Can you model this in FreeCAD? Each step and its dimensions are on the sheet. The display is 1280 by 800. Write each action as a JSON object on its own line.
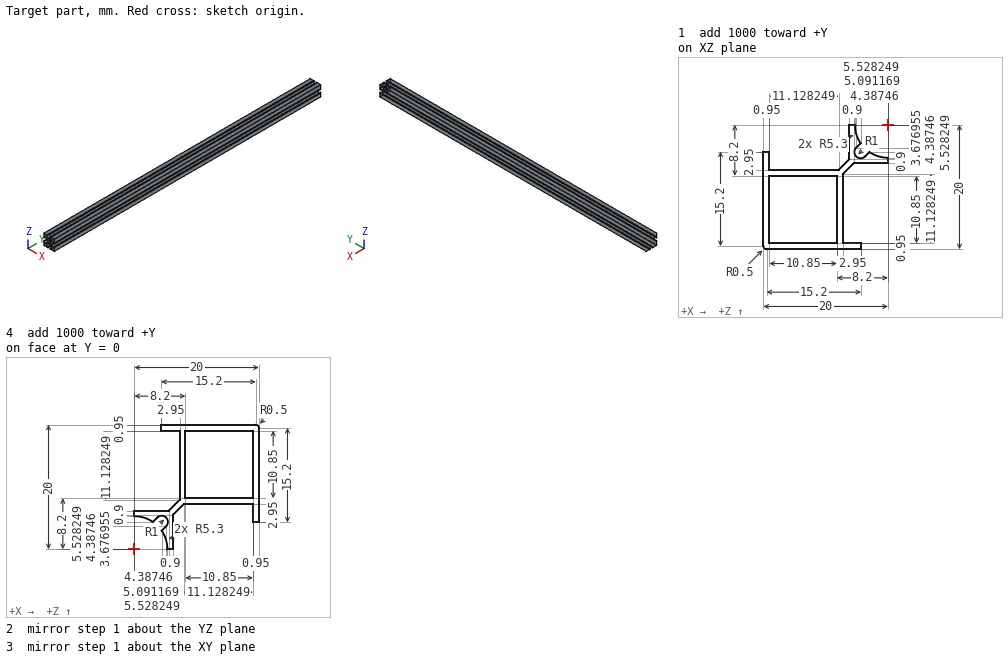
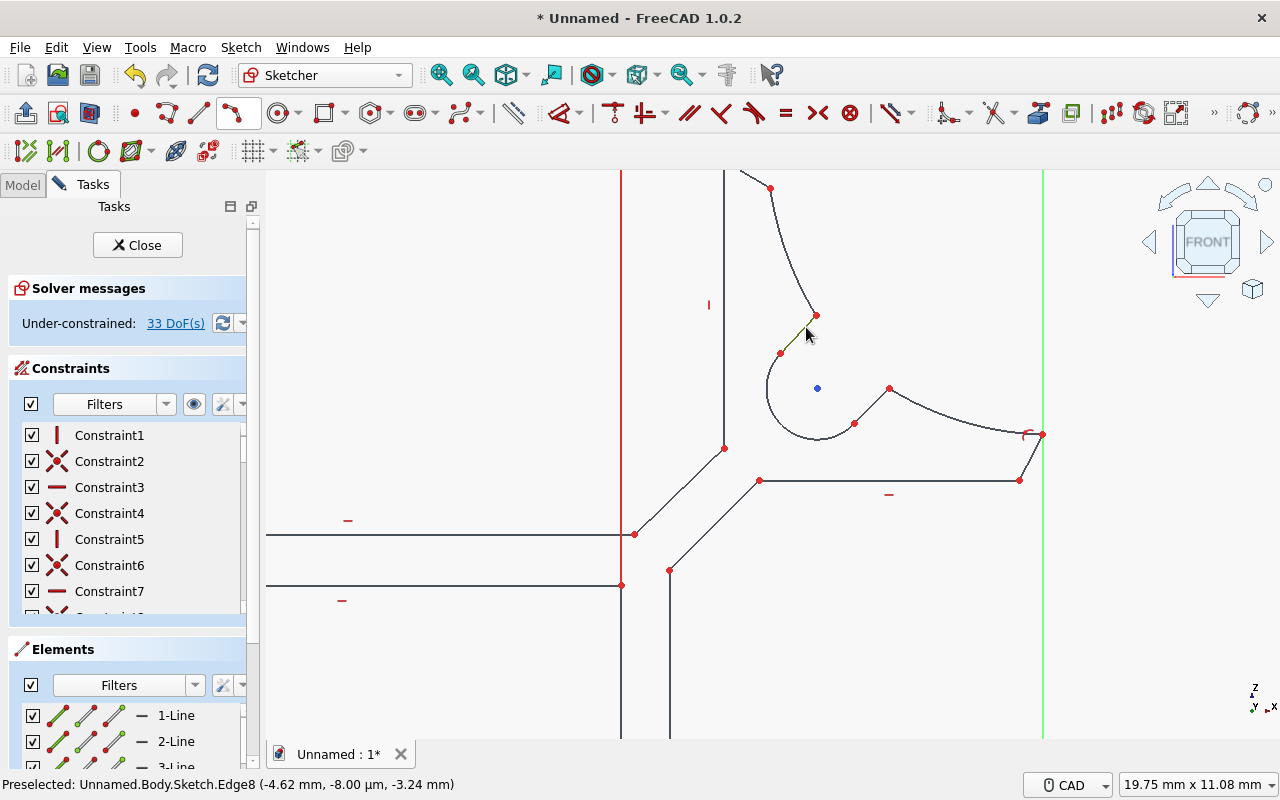
{"action": "left_click", "coordinate": [767, 398]}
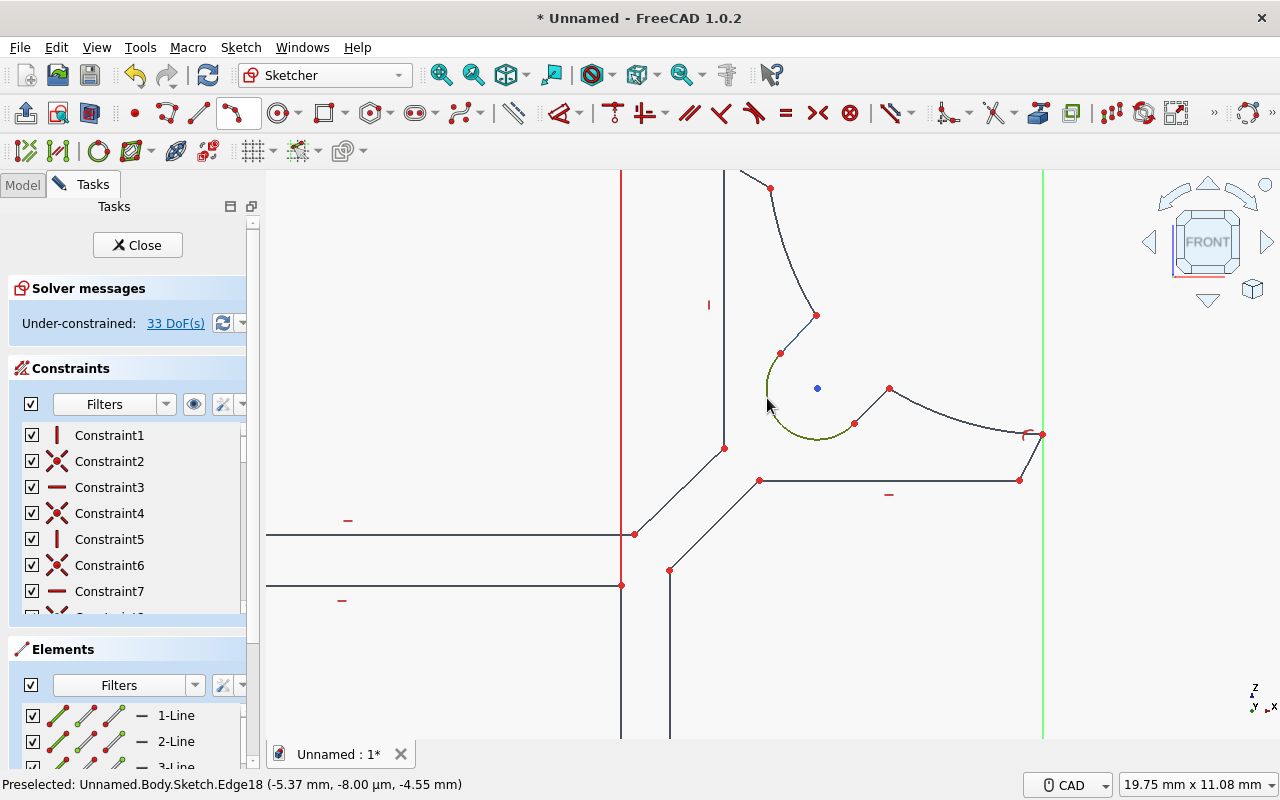
{"action": "left_click", "coordinate": [754, 114]}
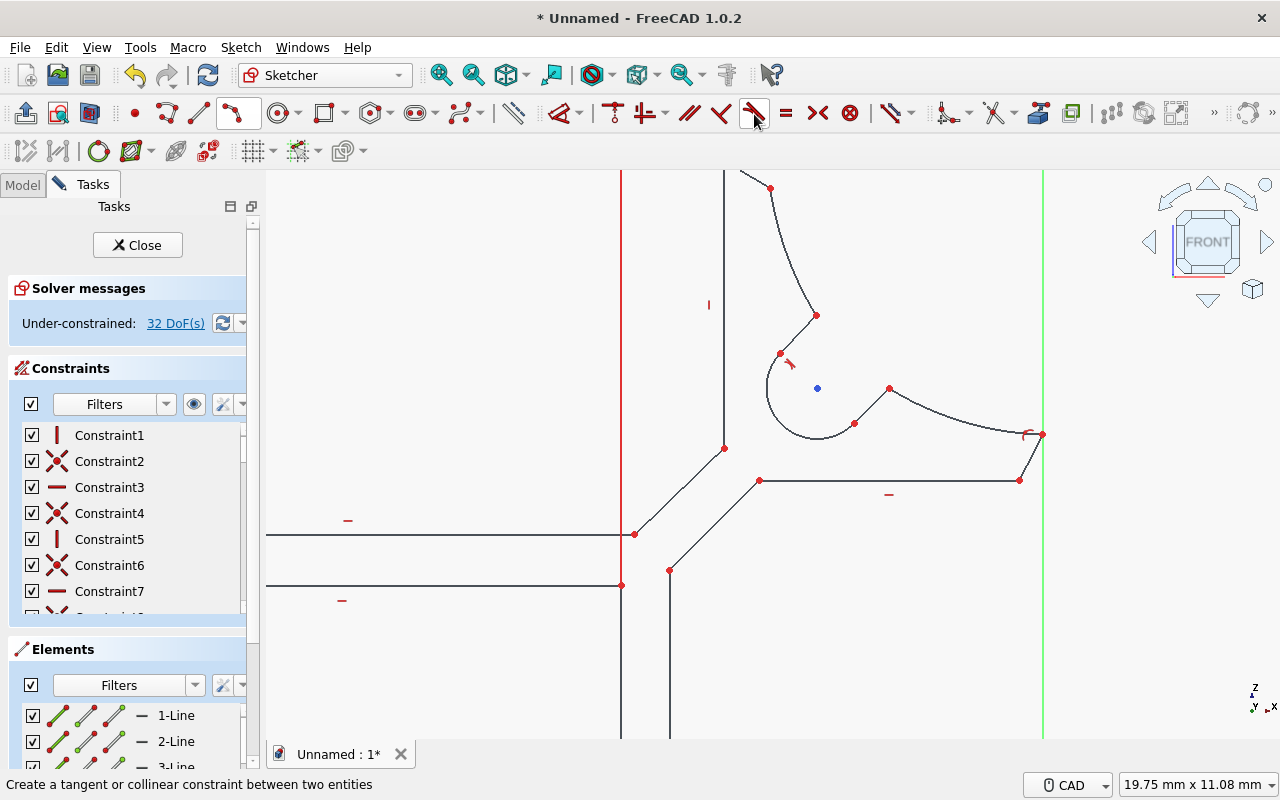
{"action": "left_click", "coordinate": [865, 413]}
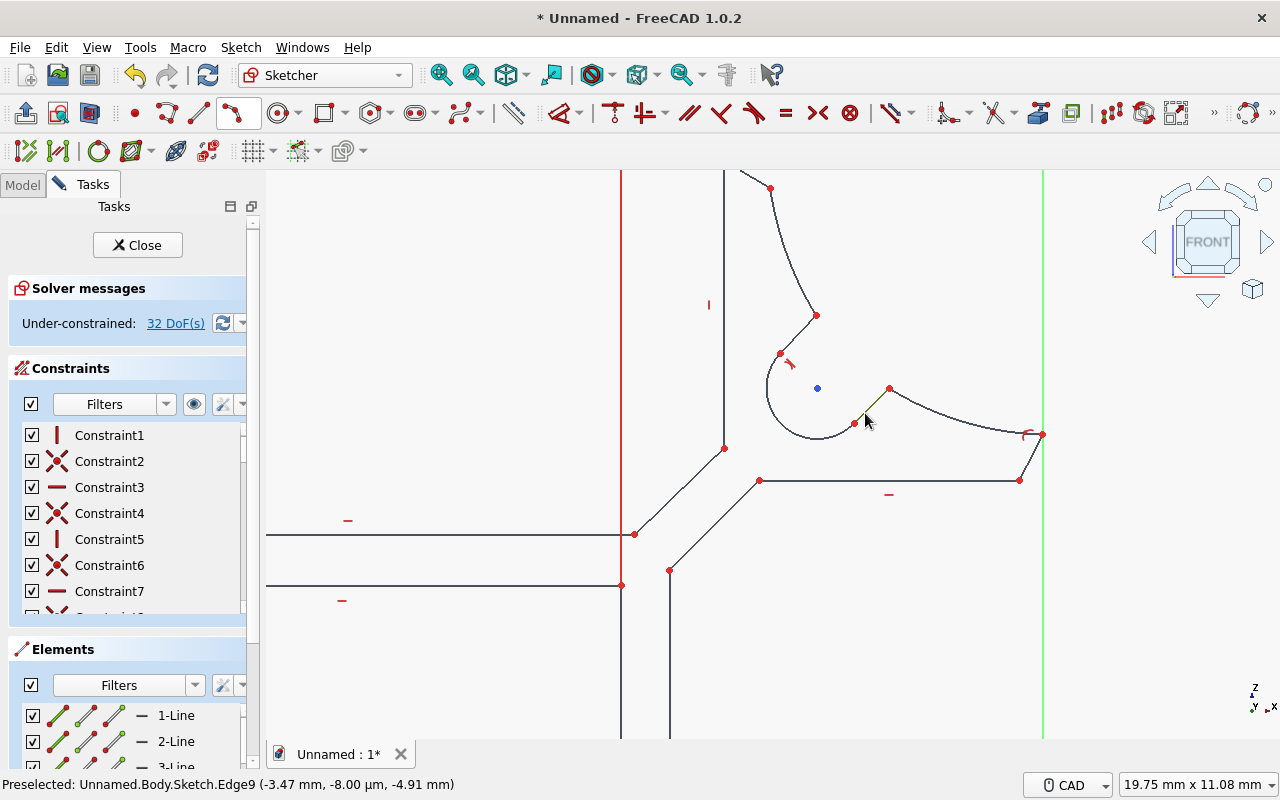
{"action": "left_click", "coordinate": [767, 398]}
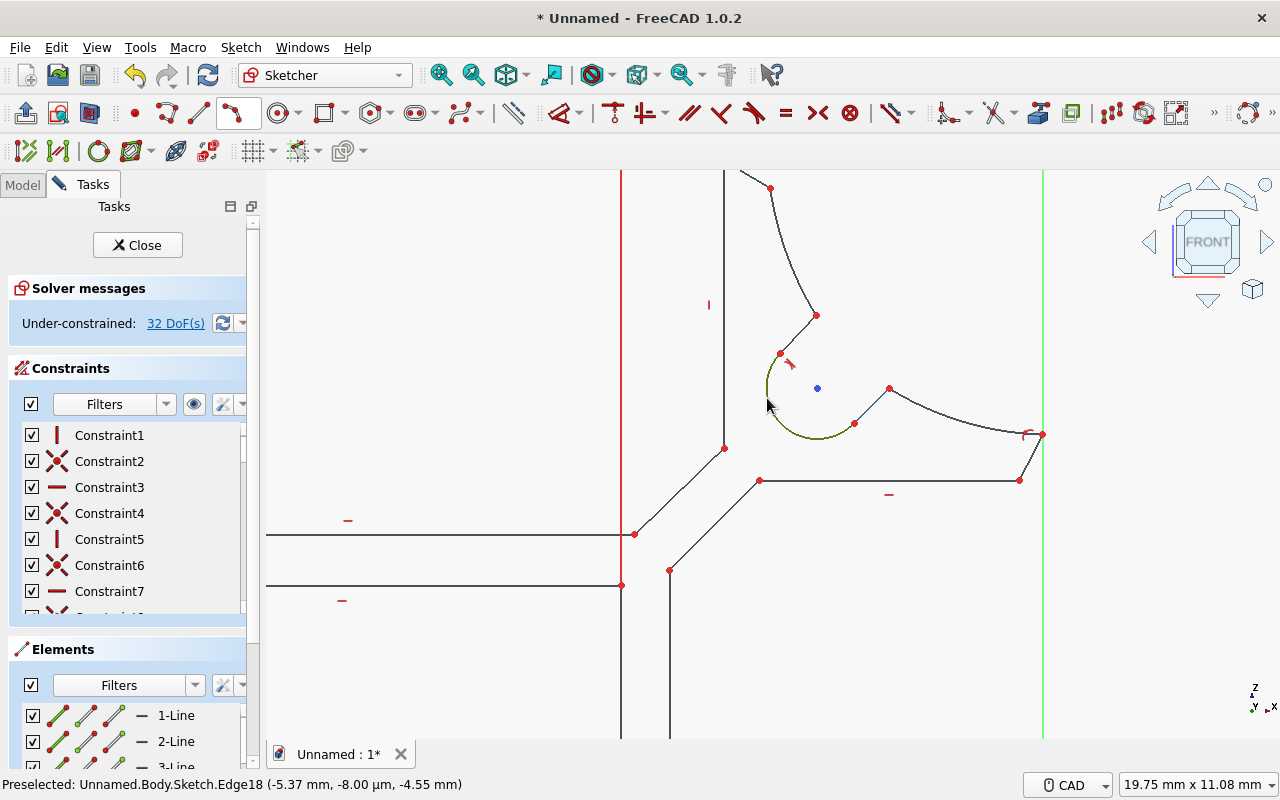
{"action": "left_click", "coordinate": [754, 114]}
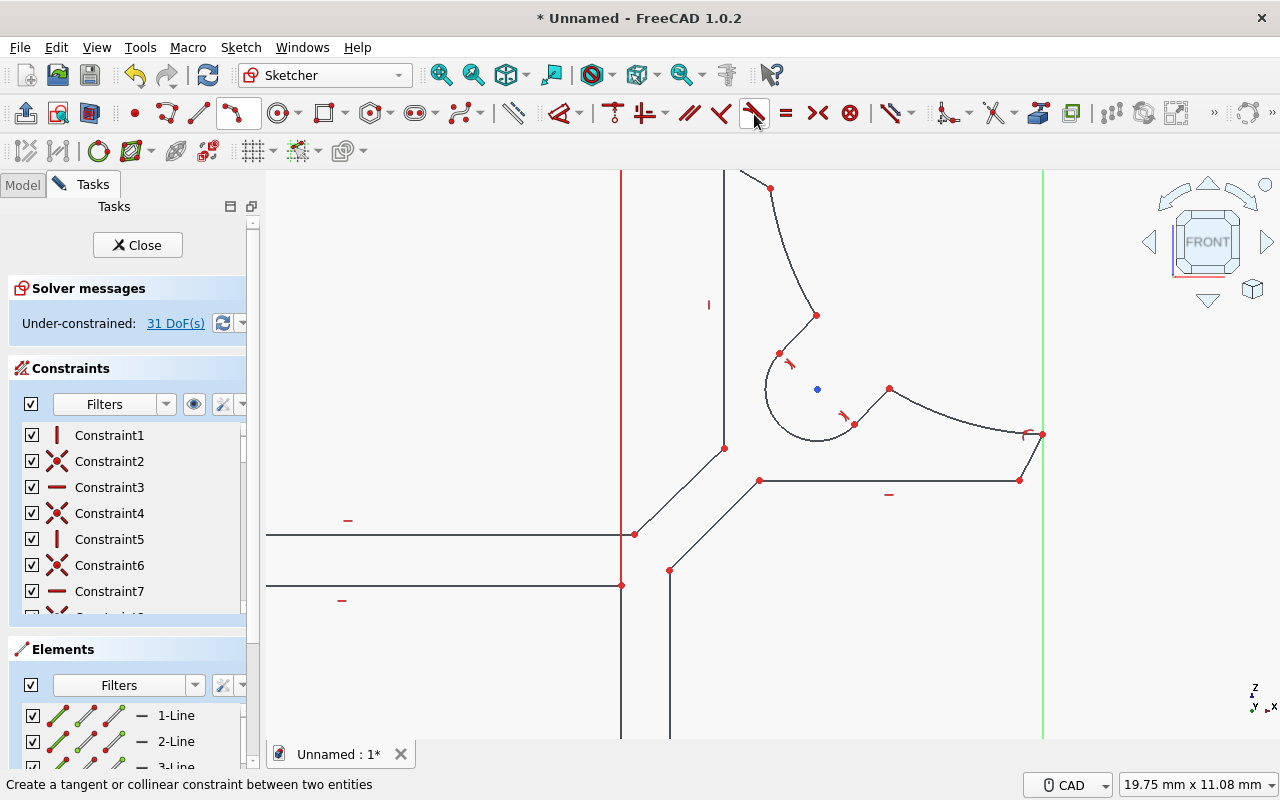
{"action": "scroll", "coordinate": [807, 327], "scroll_direction": "down", "scroll_amount": 5}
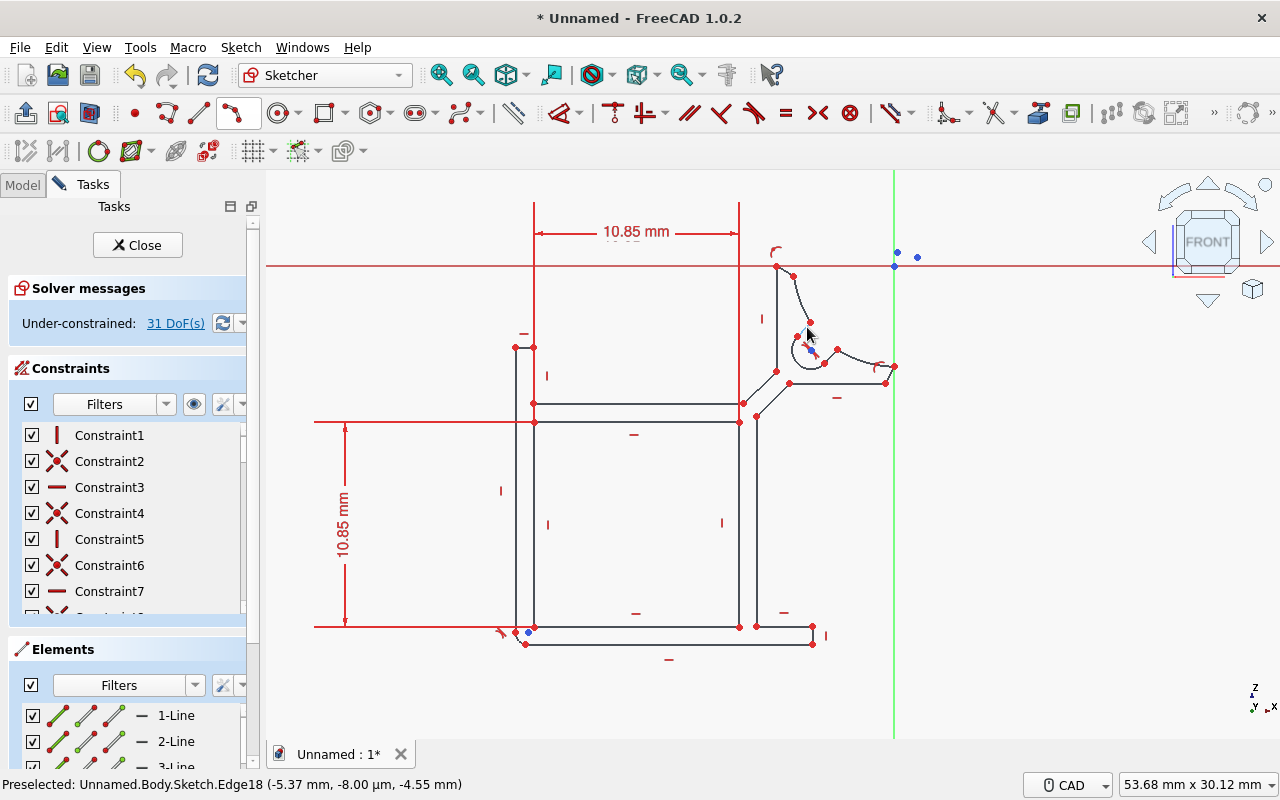
{"action": "left_click", "coordinate": [727, 645]}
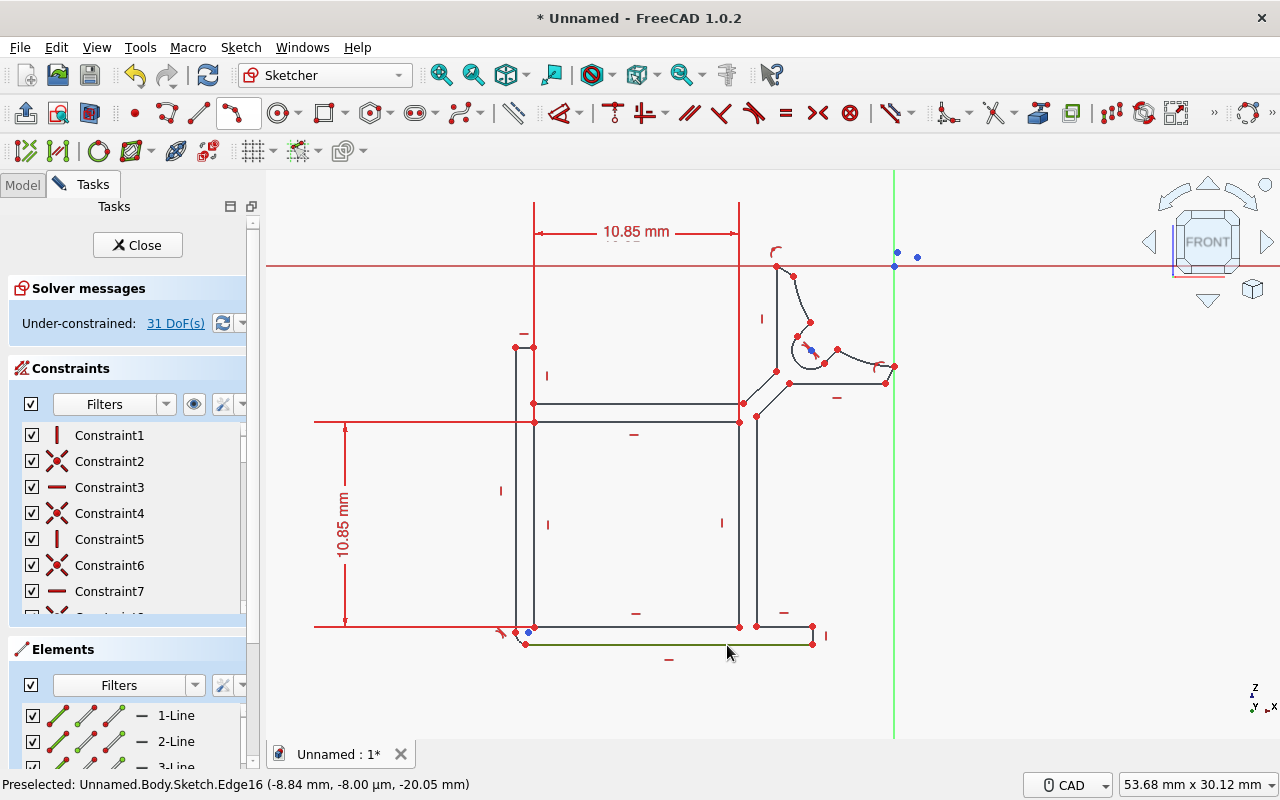
{"action": "scroll", "coordinate": [518, 641], "scroll_direction": "up", "scroll_amount": 3}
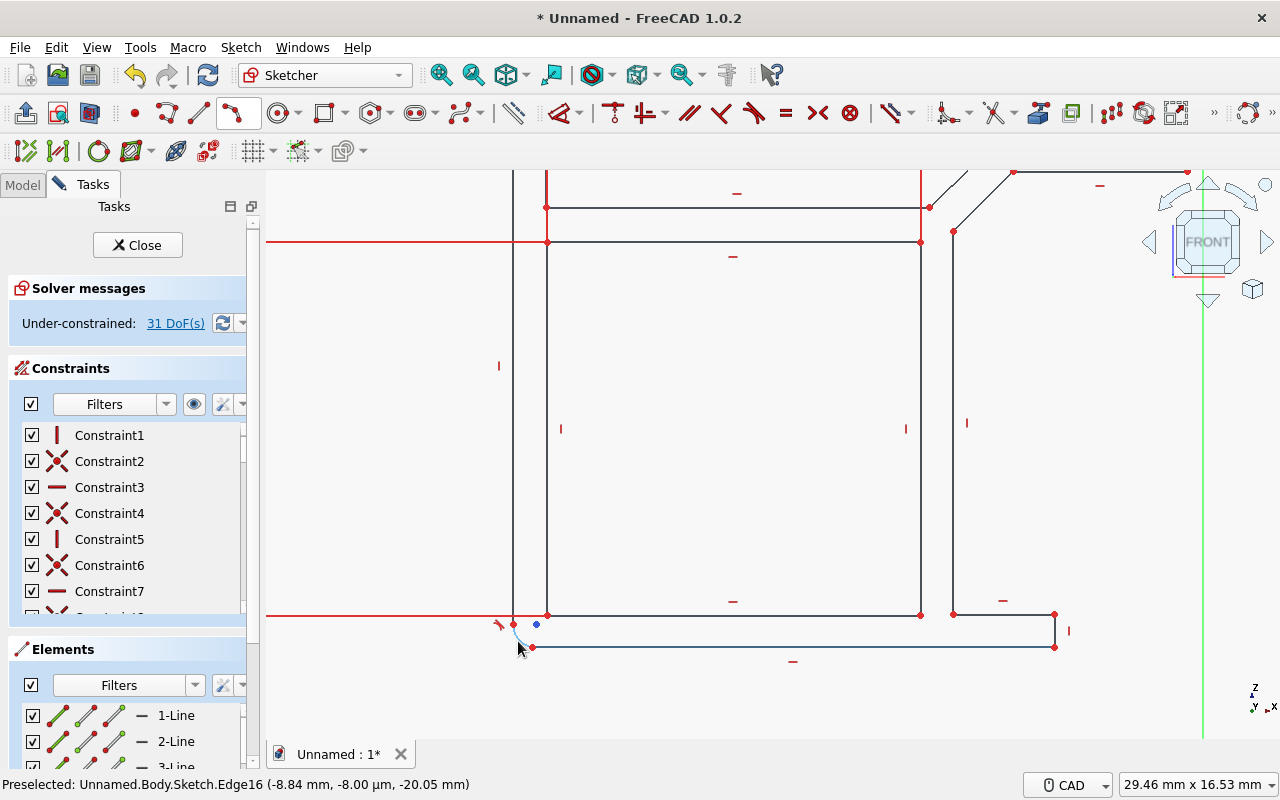
{"action": "left_click", "coordinate": [519, 639]}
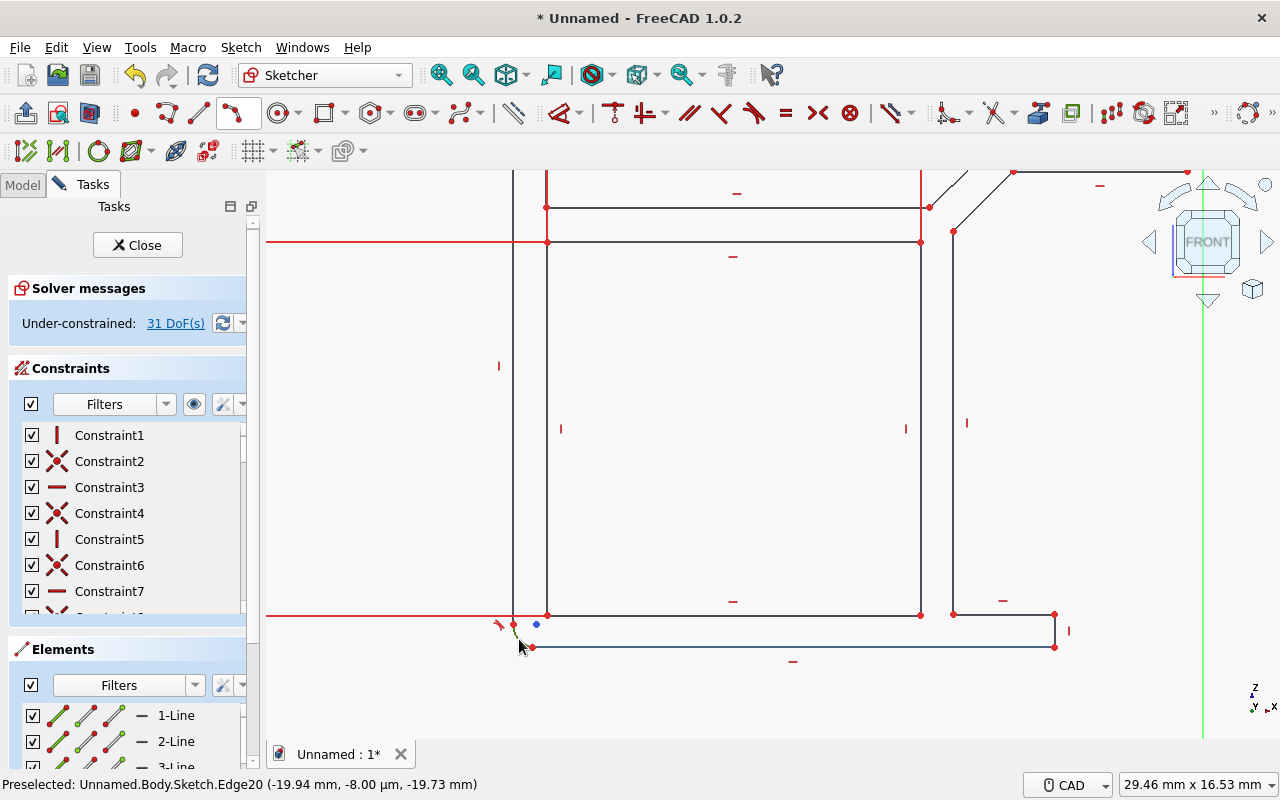
{"action": "key", "text": "t"}